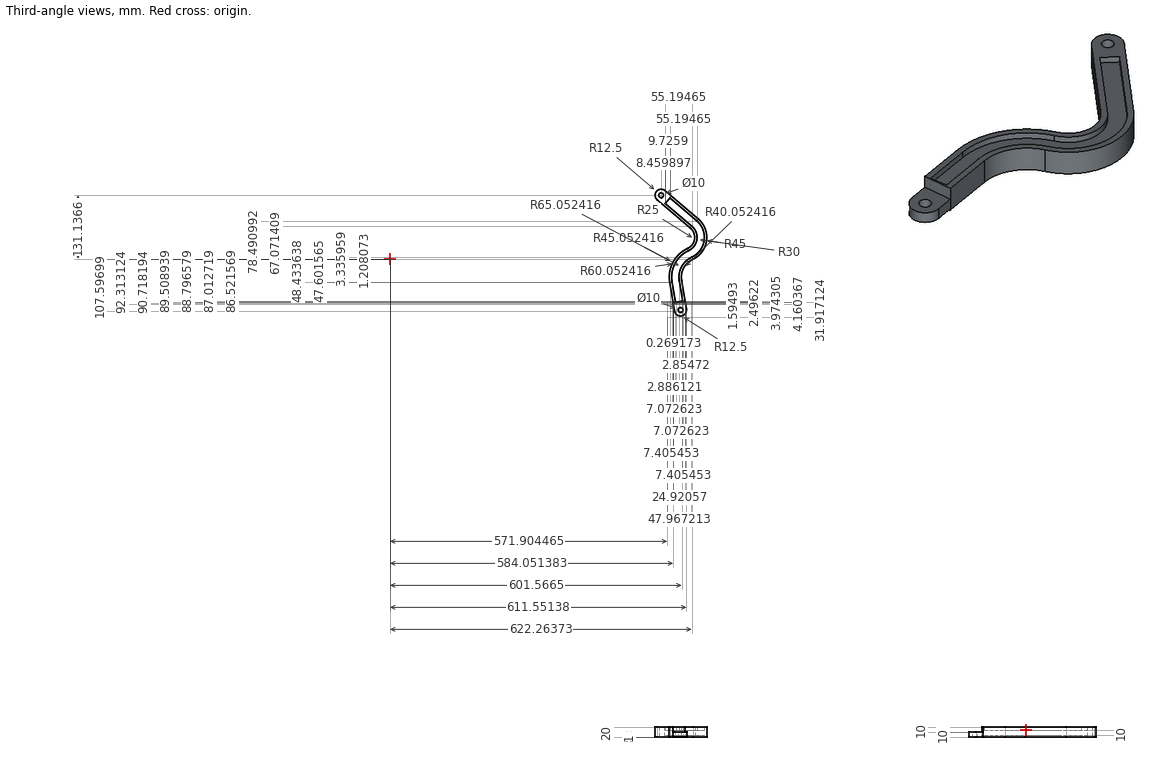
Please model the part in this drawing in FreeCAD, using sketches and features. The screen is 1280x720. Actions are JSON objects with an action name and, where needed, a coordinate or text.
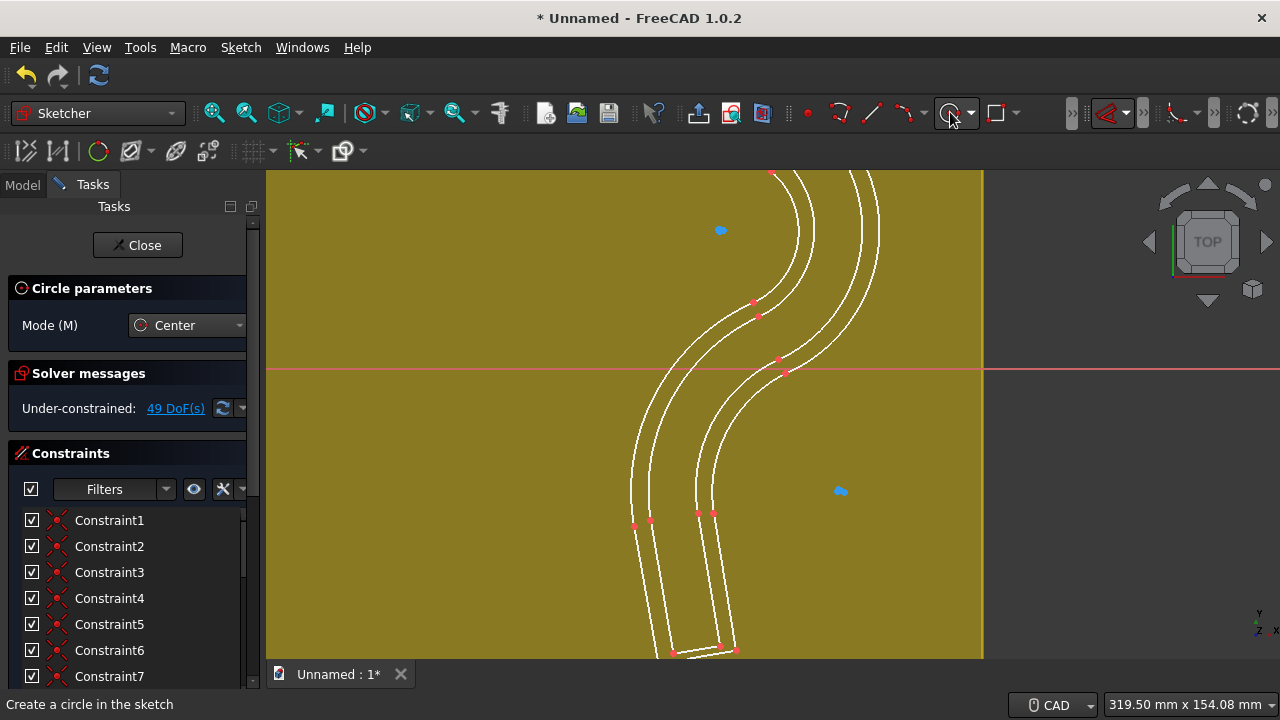
{"action": "scroll", "coordinate": [698, 514], "scroll_direction": "down", "scroll_amount": 4}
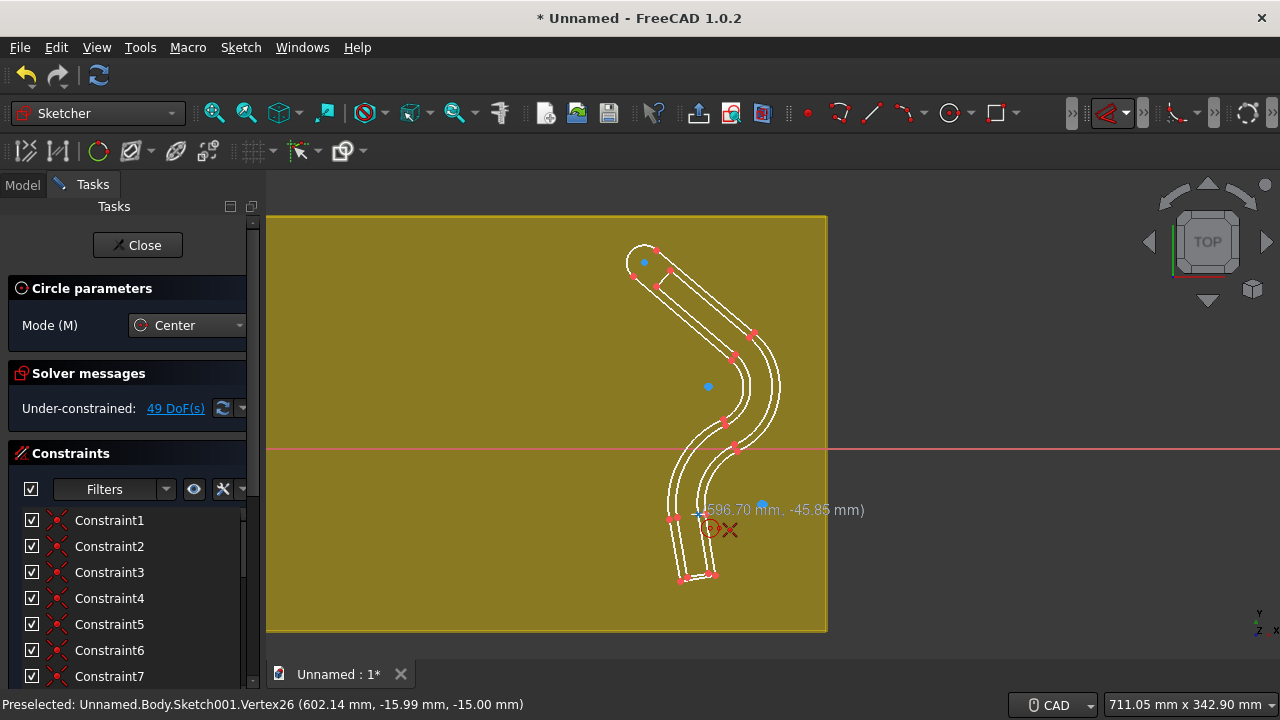
{"action": "scroll", "coordinate": [645, 262], "scroll_direction": "up", "scroll_amount": 6}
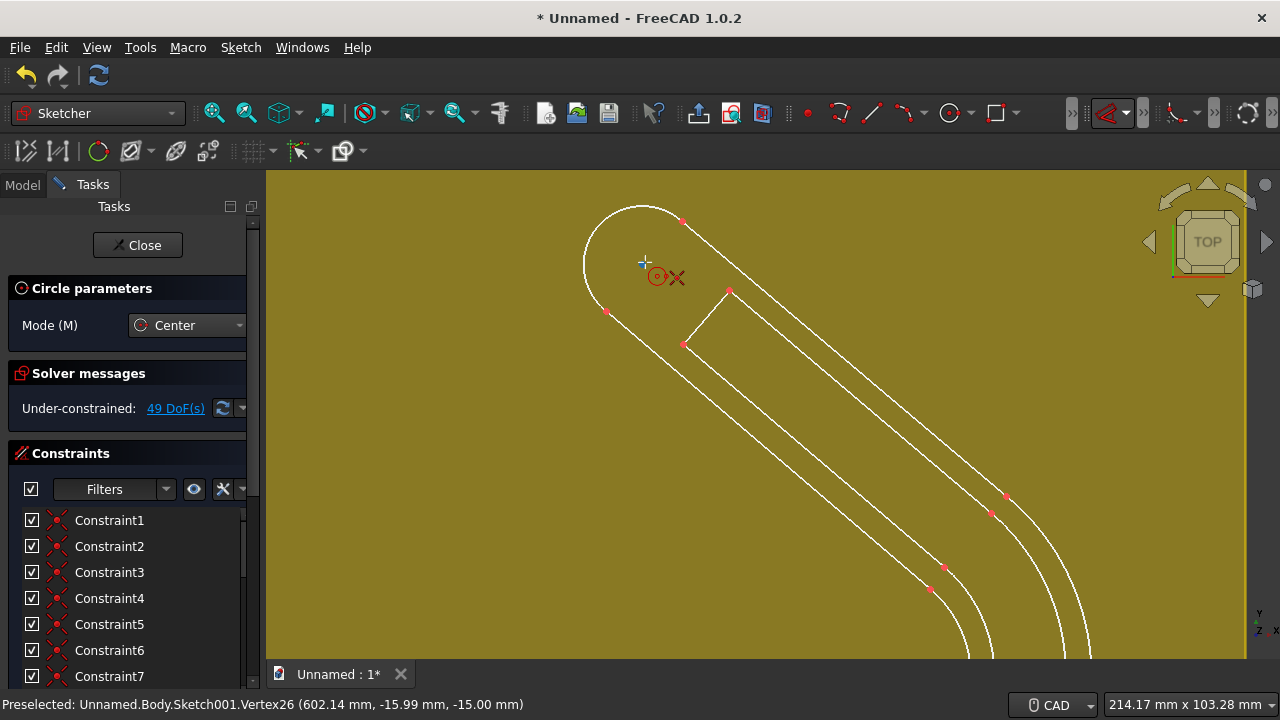
{"action": "left_click", "coordinate": [644, 263]}
{"action": "left_click", "coordinate": [660, 246]}
{"action": "key", "text": "Escape"}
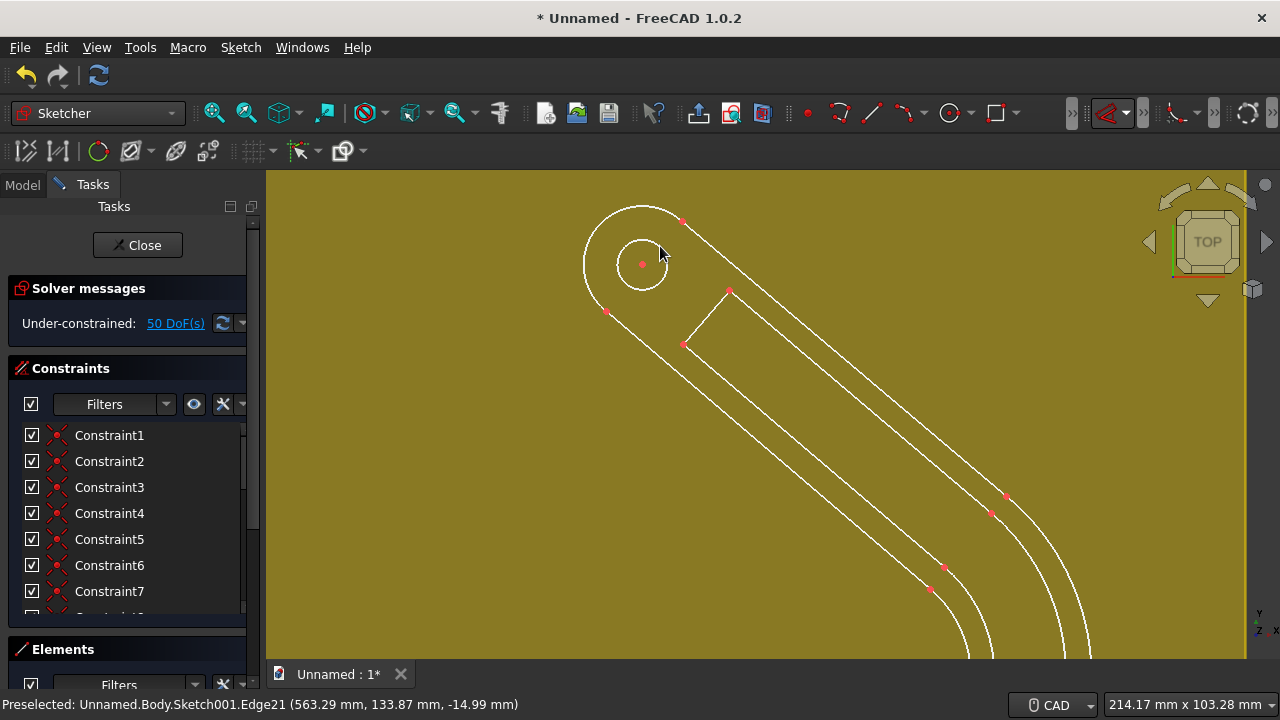
{"action": "left_click", "coordinate": [909, 414]}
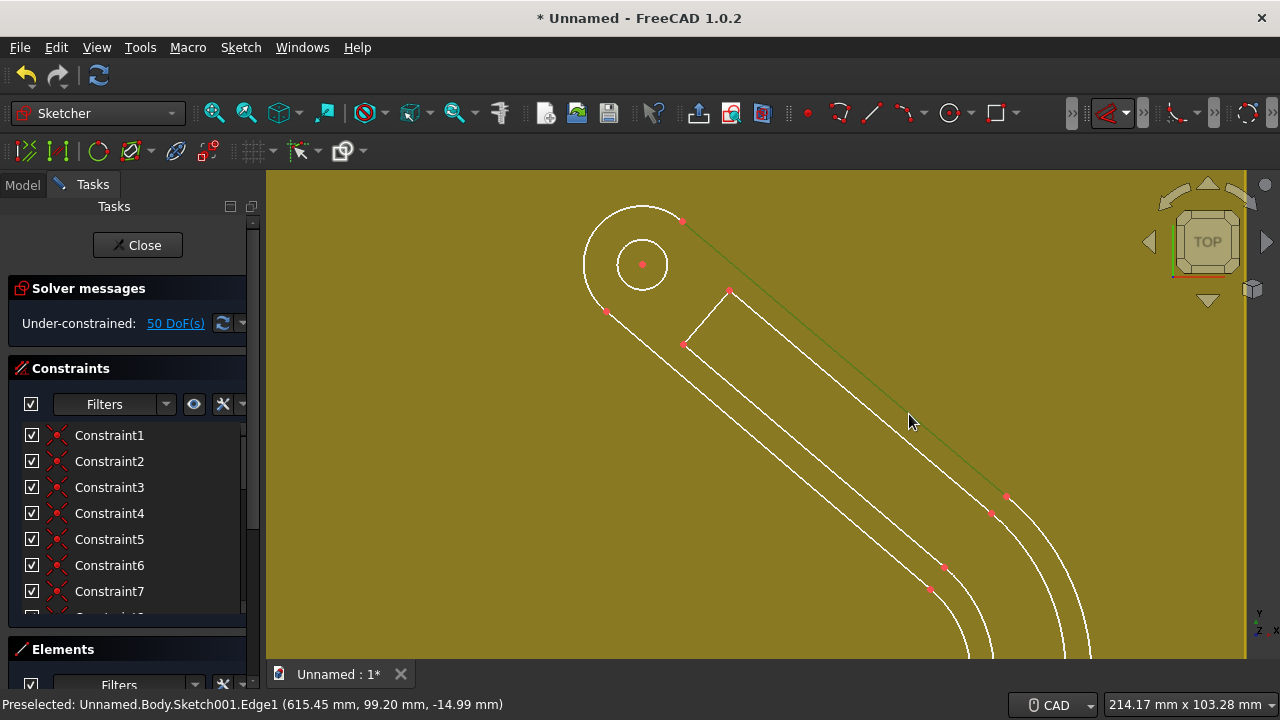
{"action": "left_click", "coordinate": [630, 207]}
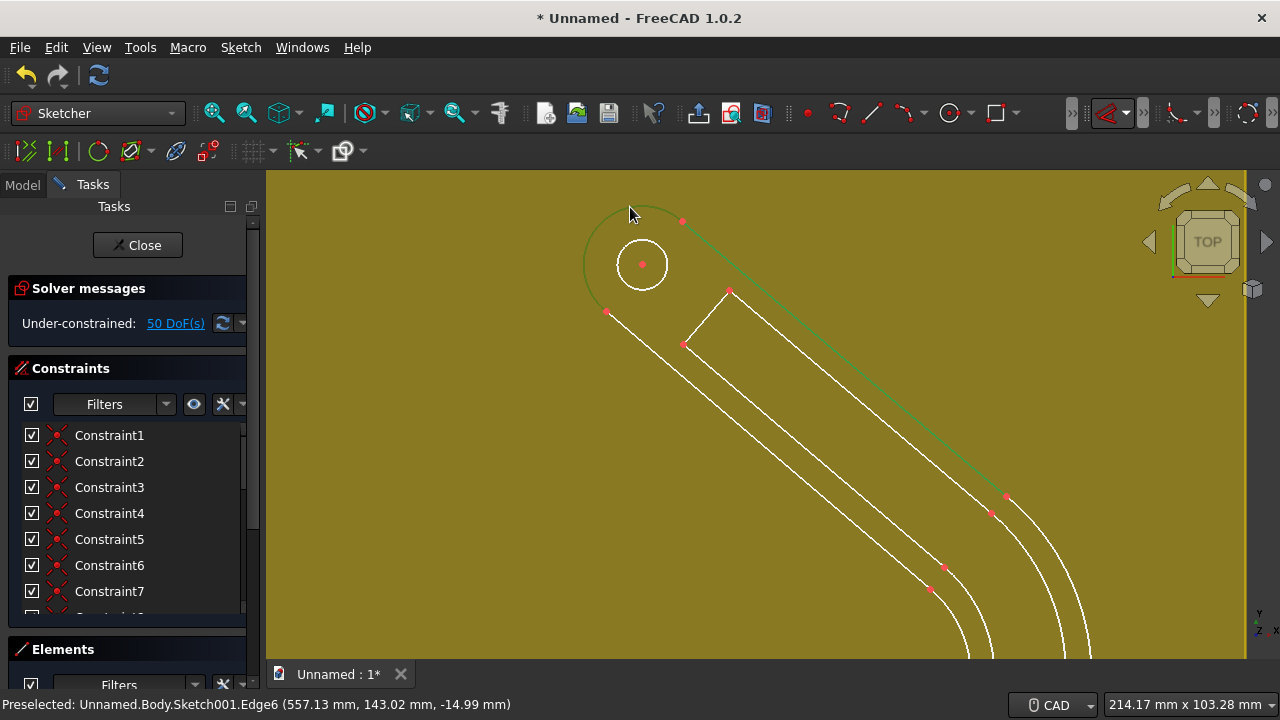
{"action": "key", "text": "t"}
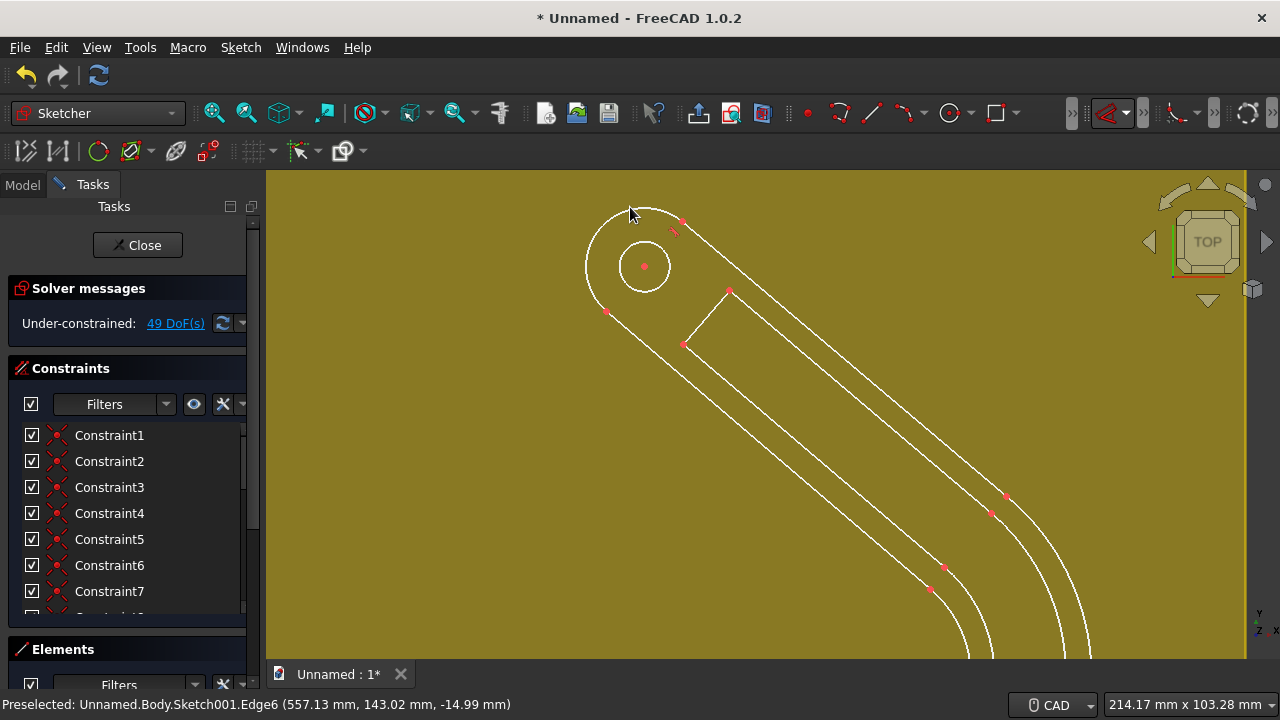
{"action": "left_click", "coordinate": [909, 414]}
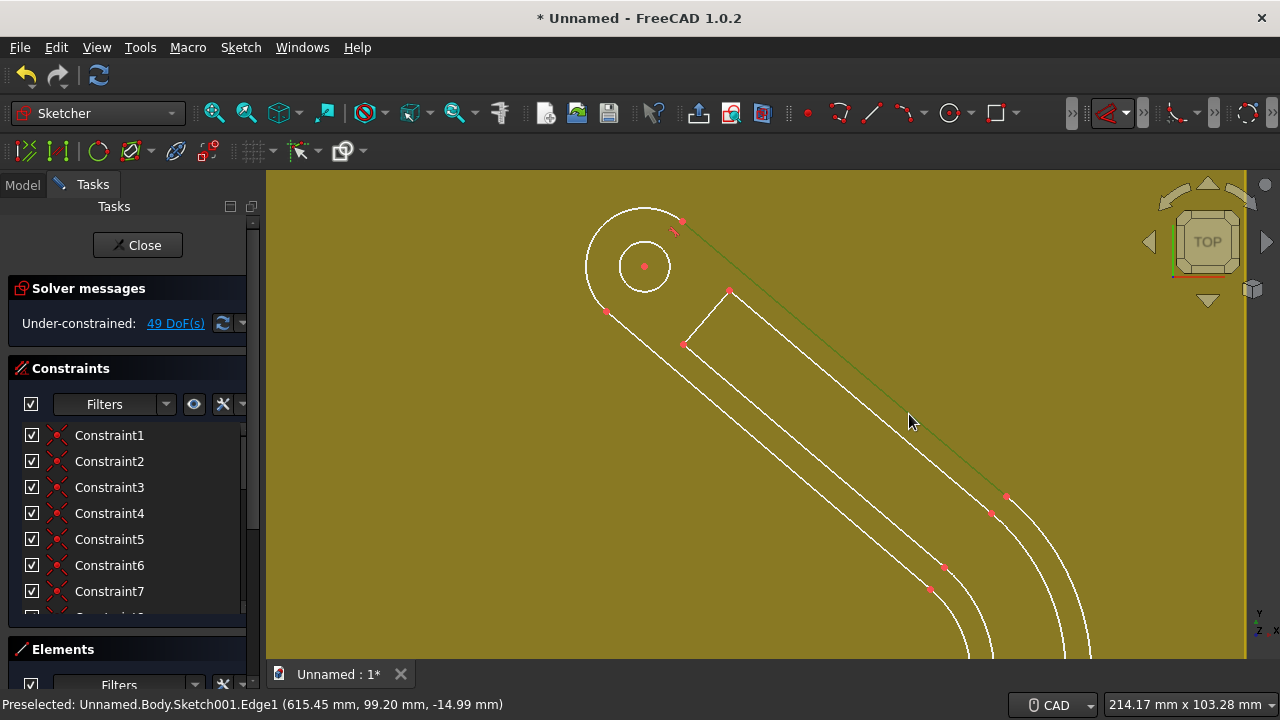
{"action": "left_click", "coordinate": [1083, 614]}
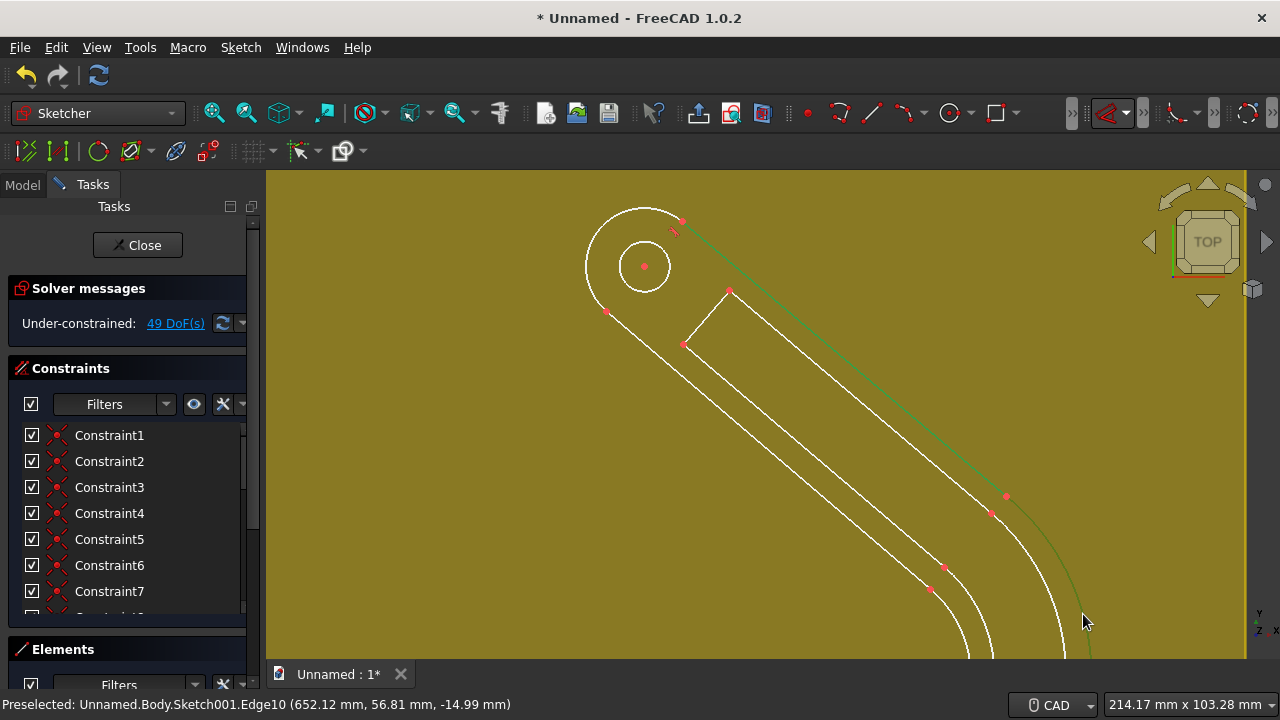
{"action": "key", "text": "t"}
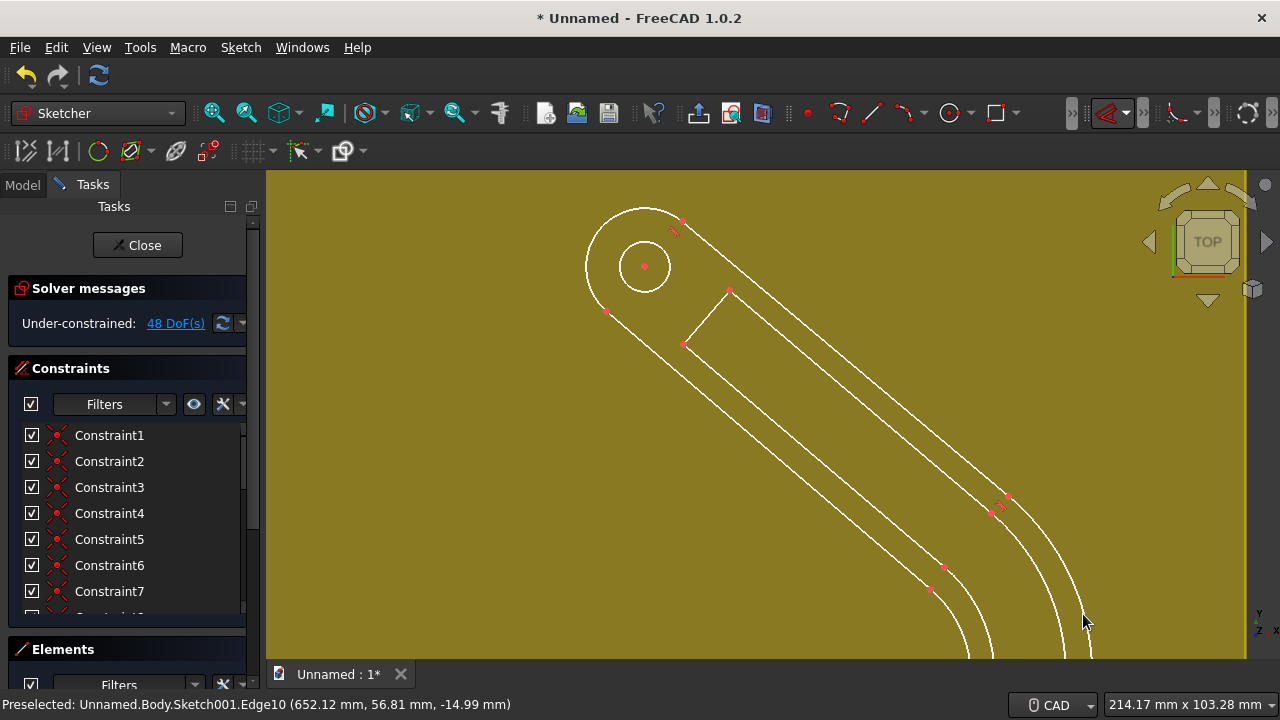
{"action": "left_click", "coordinate": [704, 395]}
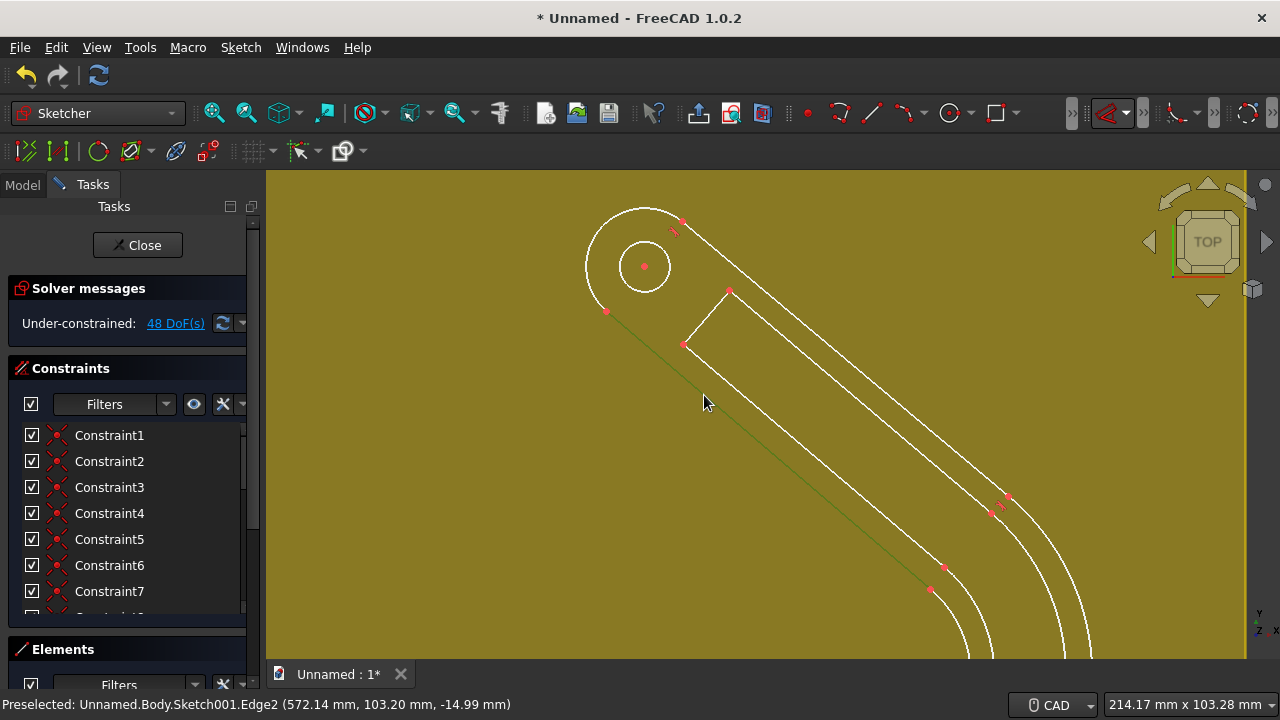
{"action": "left_click", "coordinate": [631, 210]}